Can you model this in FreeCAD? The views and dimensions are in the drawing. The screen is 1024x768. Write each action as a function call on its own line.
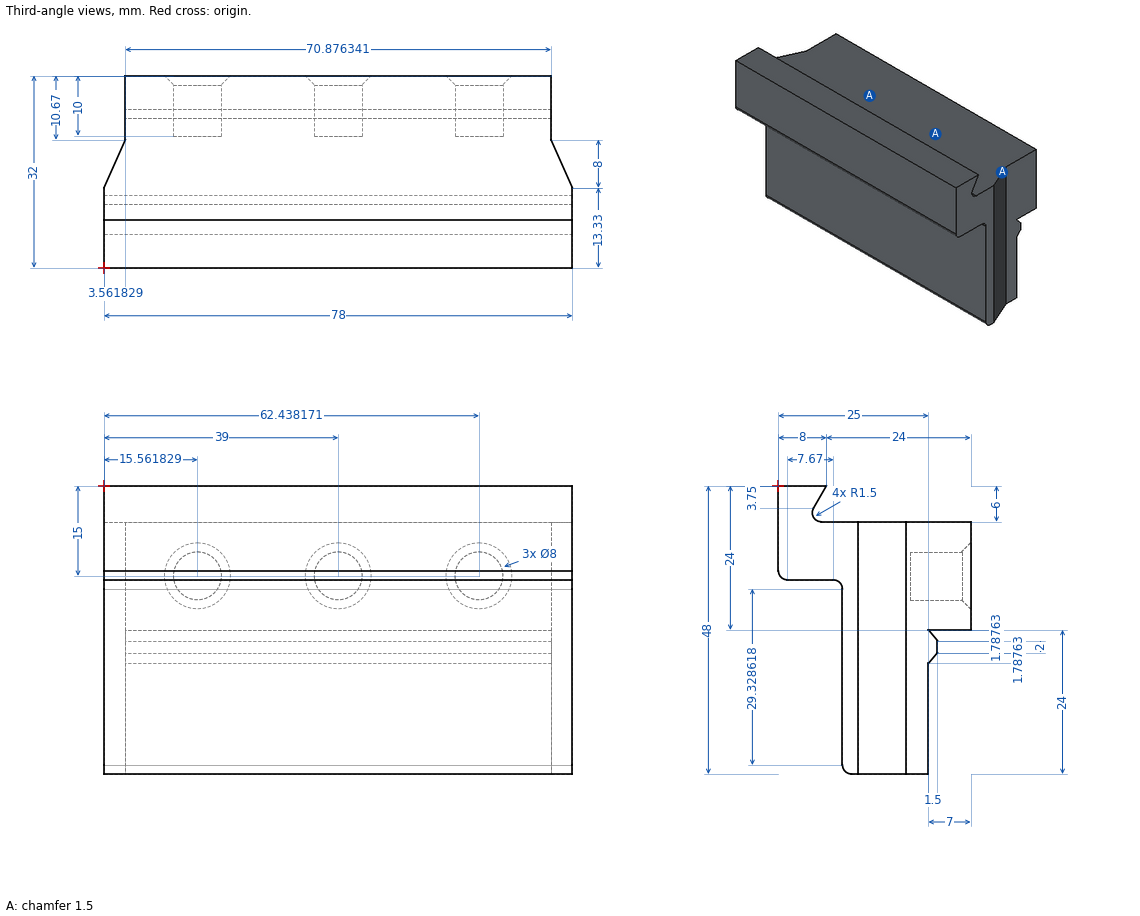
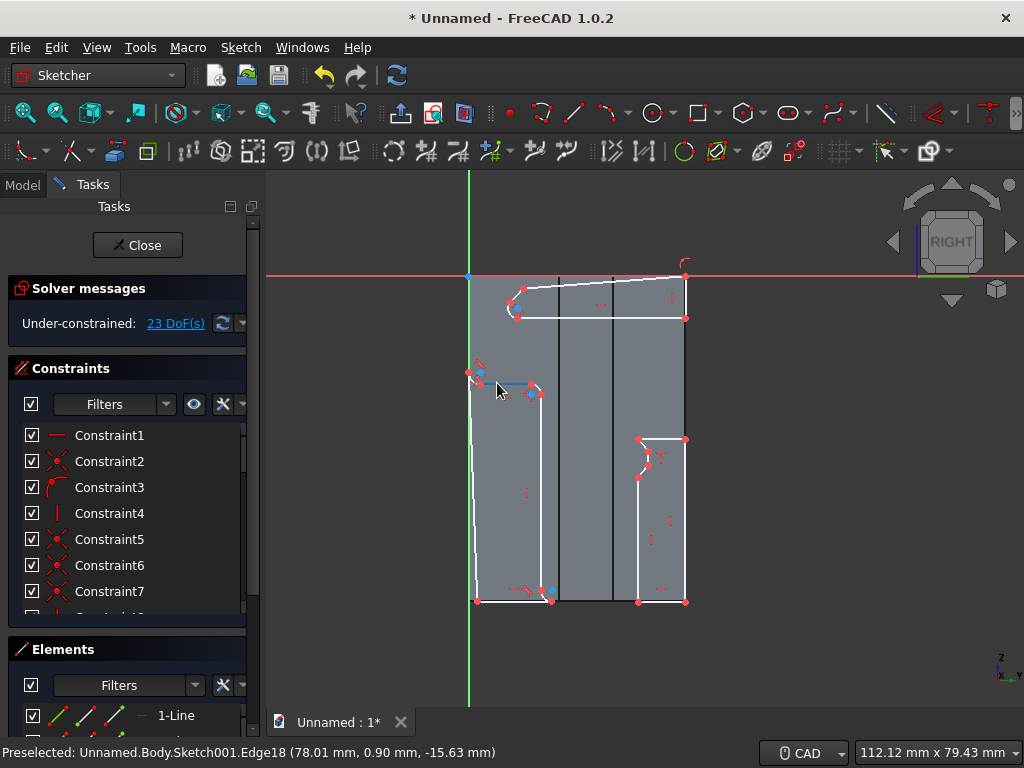
click(500, 602)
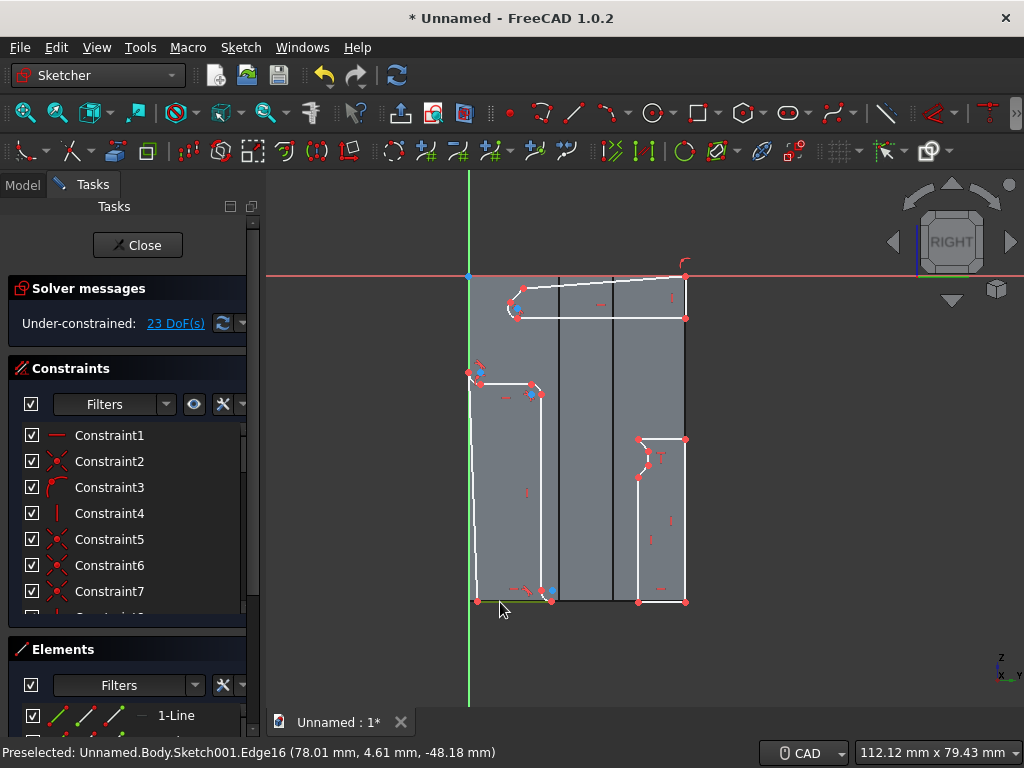
scroll(542, 596, up, 6)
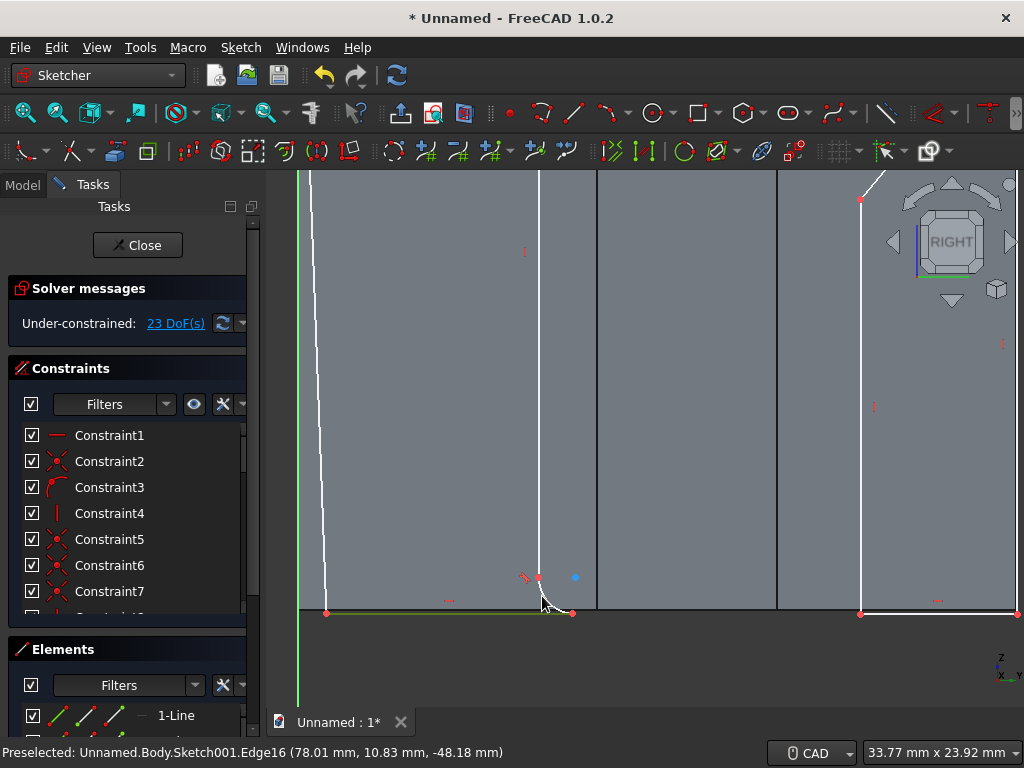
click(542, 593)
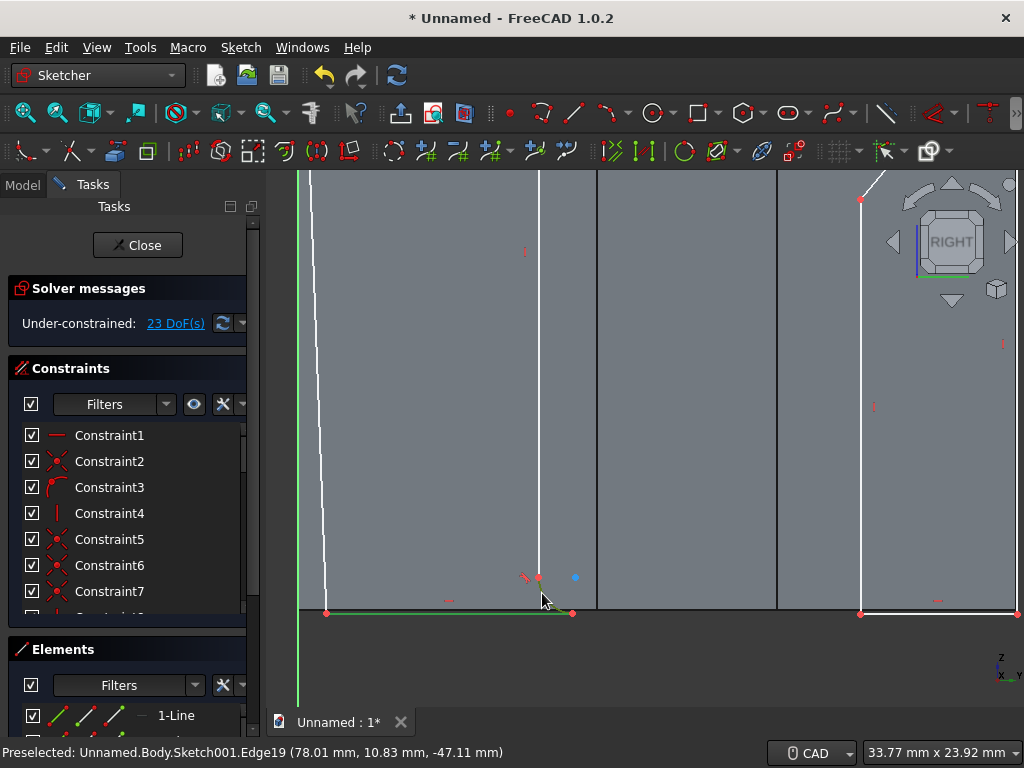
key(t)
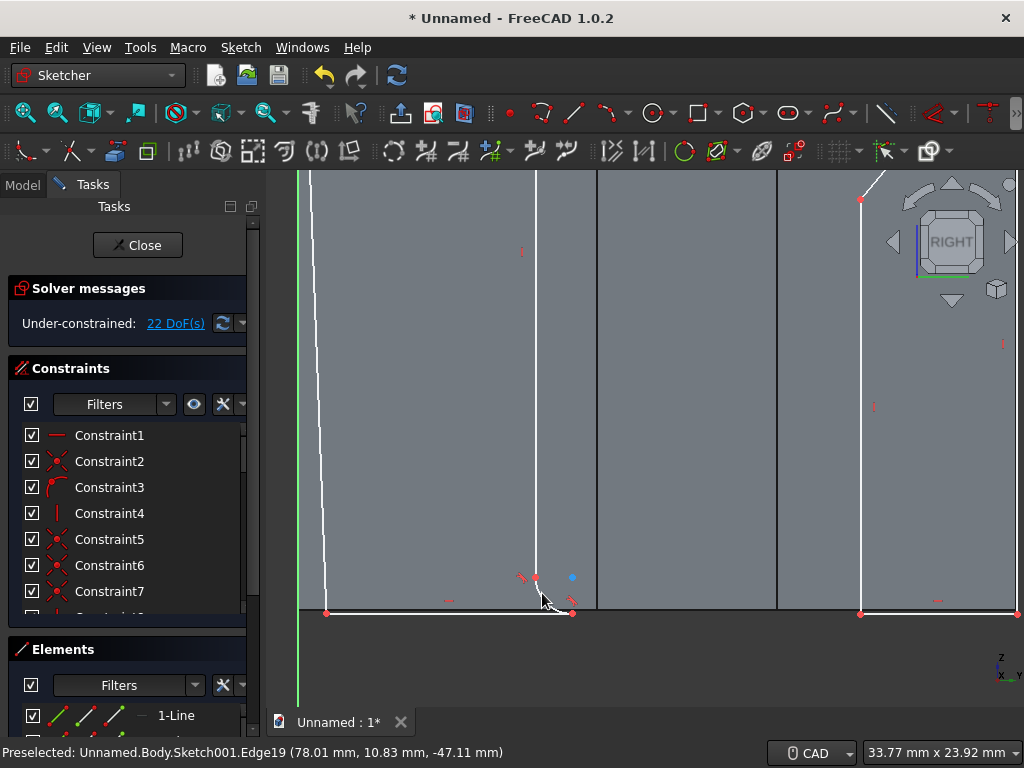
scroll(542, 597, down, 6)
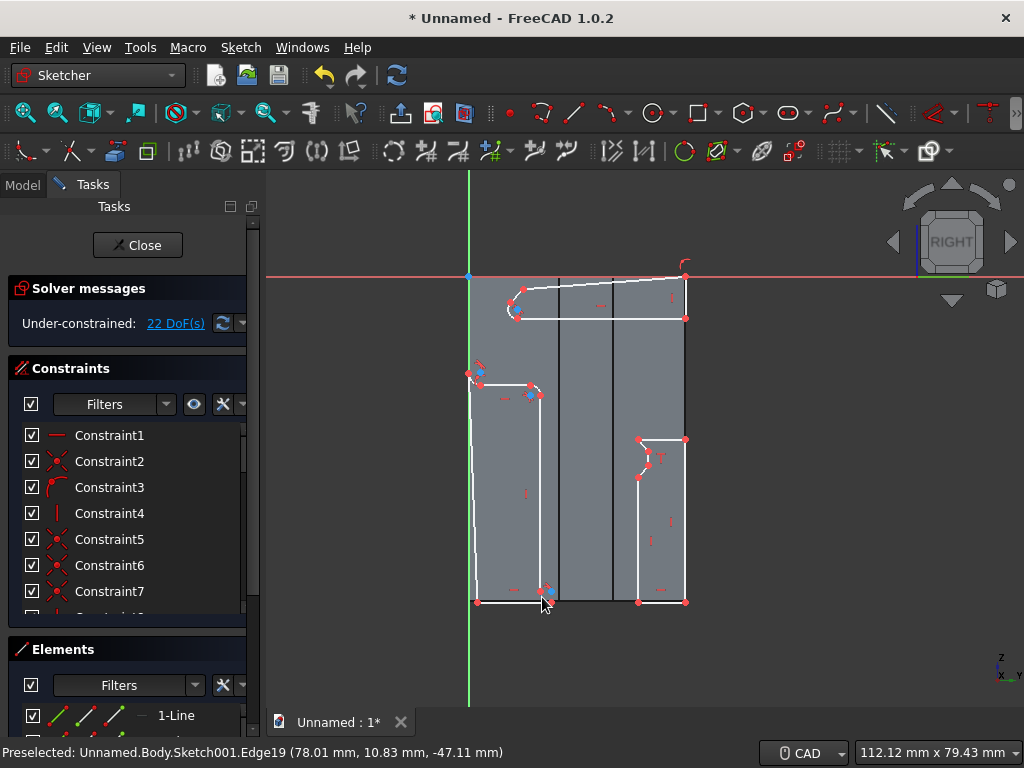
scroll(637, 281, up, 7)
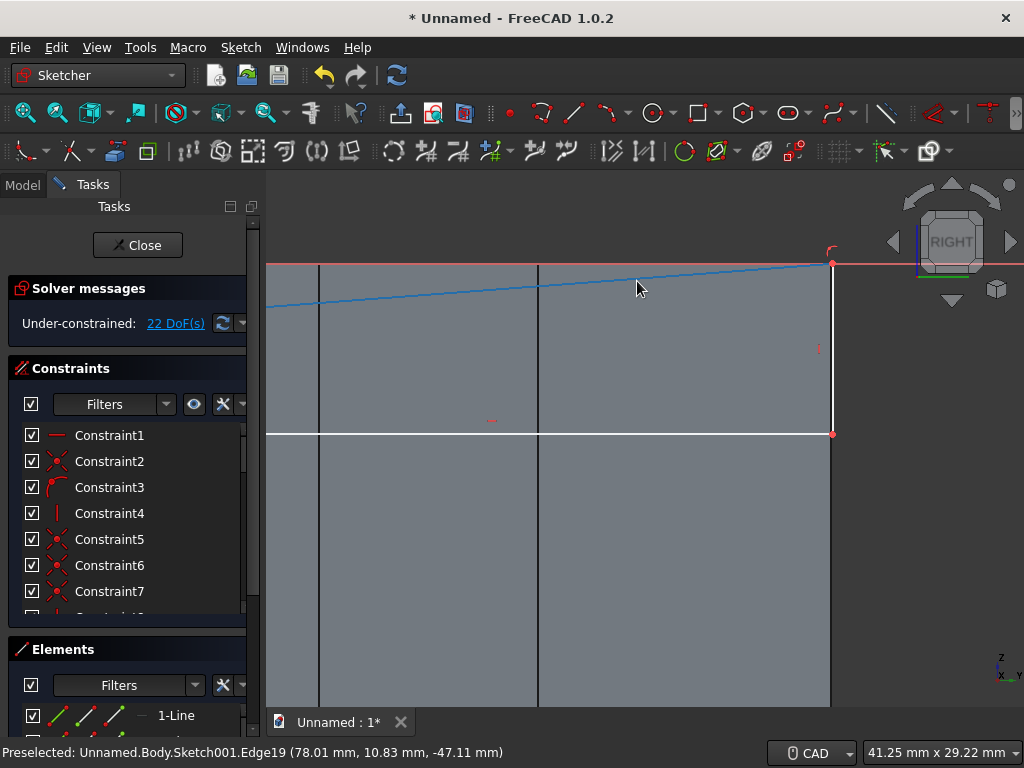
click(635, 279)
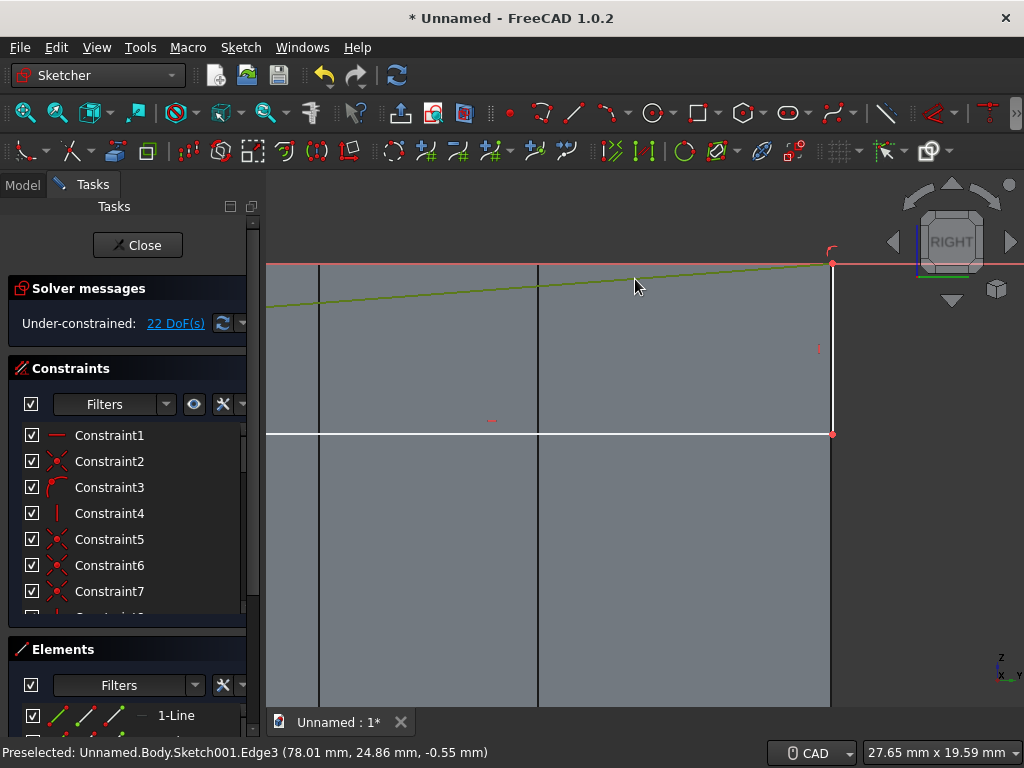
key(h)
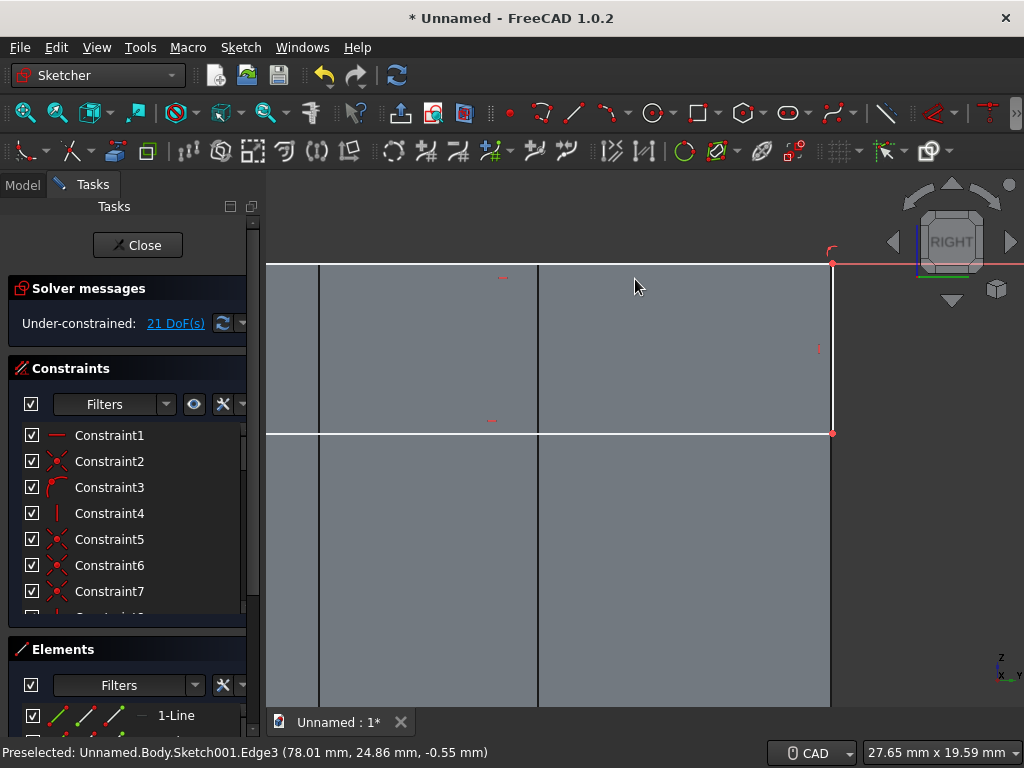
scroll(637, 280, down, 7)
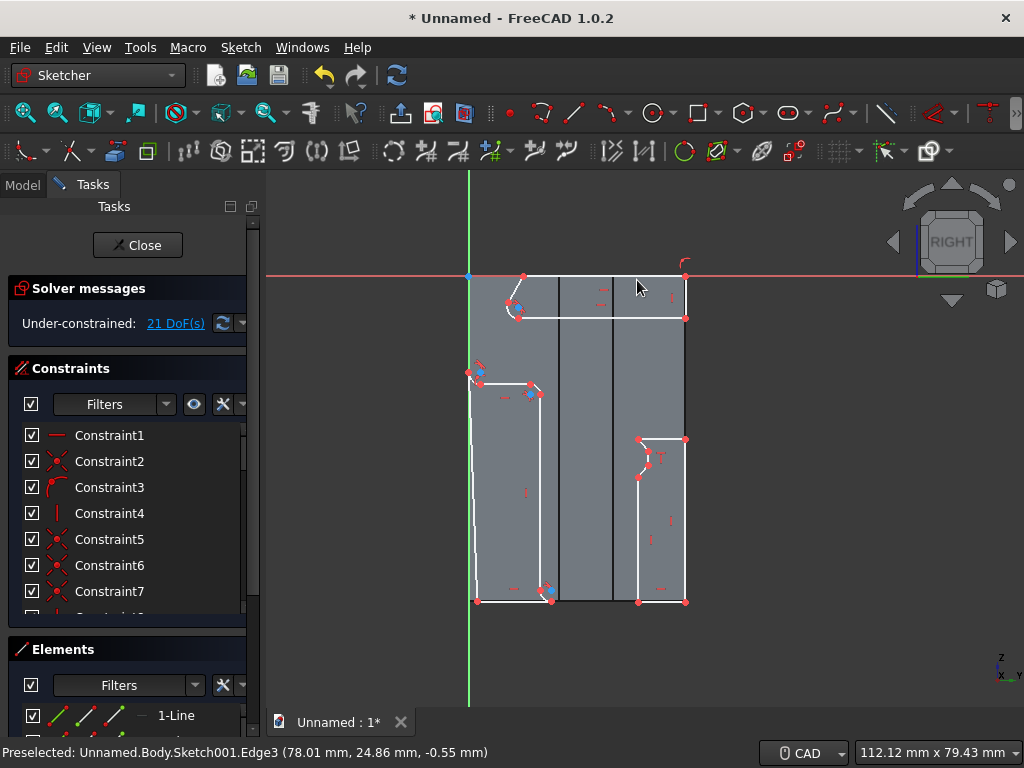
scroll(471, 441, up, 9)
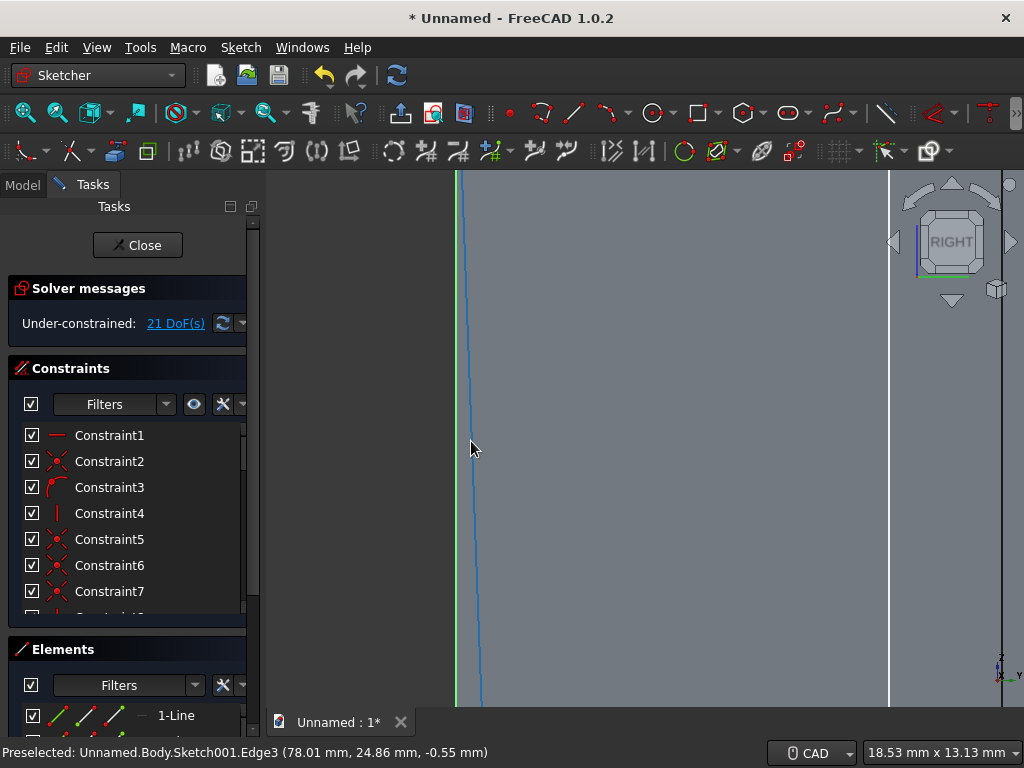
click(472, 441)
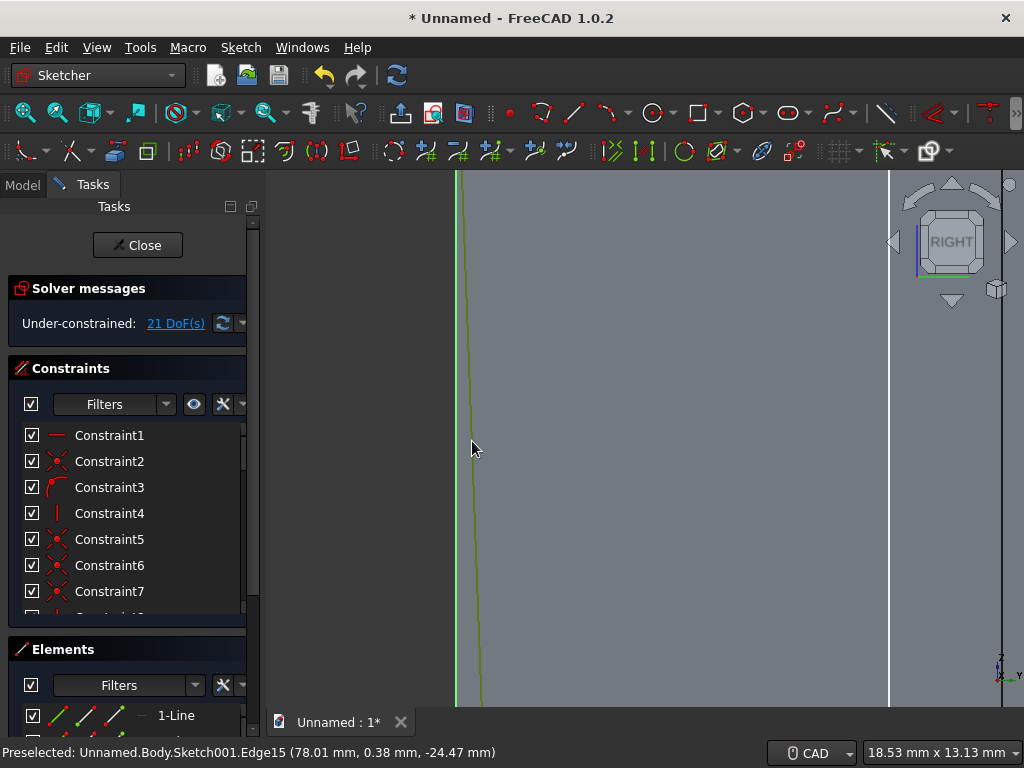
key(v)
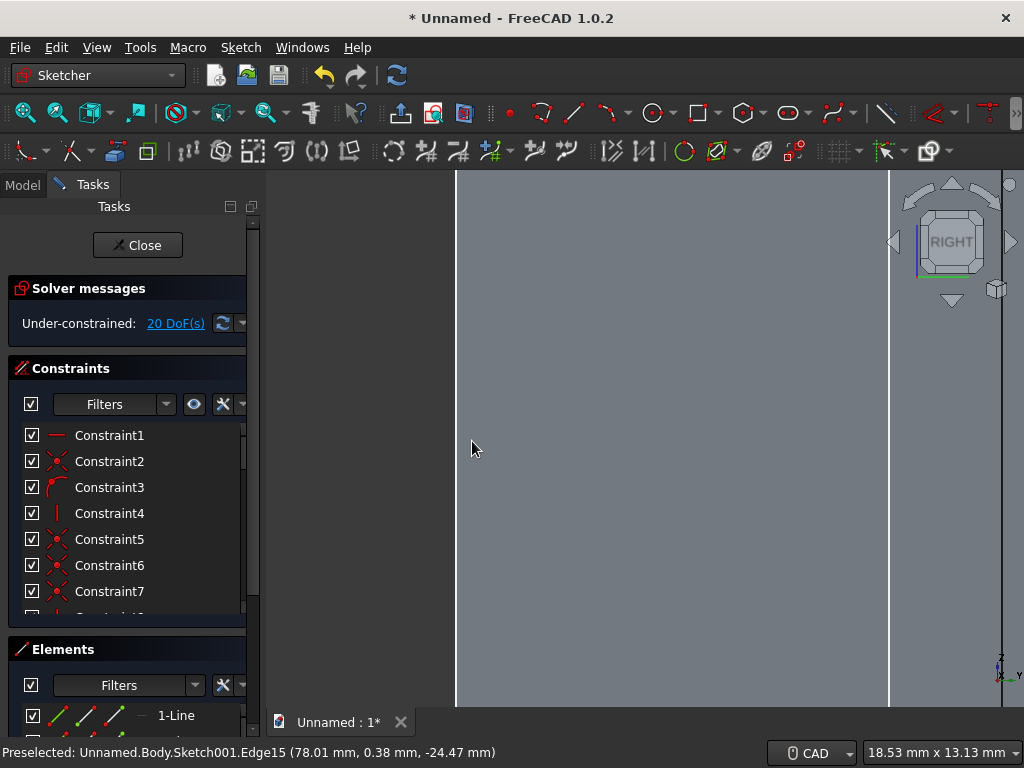
scroll(471, 442, down, 9)